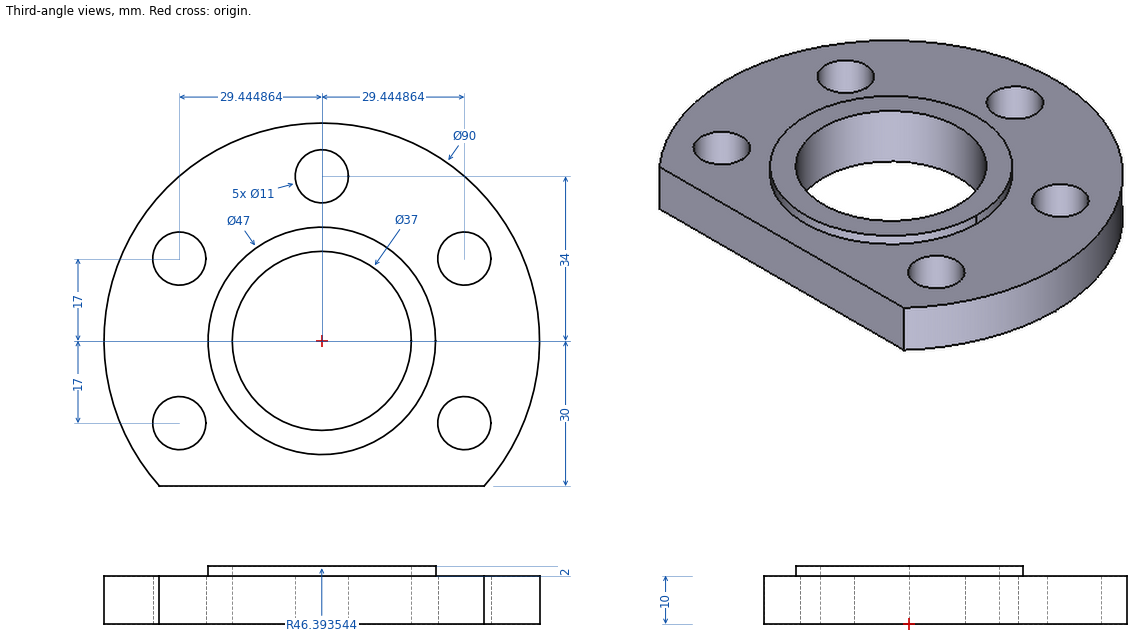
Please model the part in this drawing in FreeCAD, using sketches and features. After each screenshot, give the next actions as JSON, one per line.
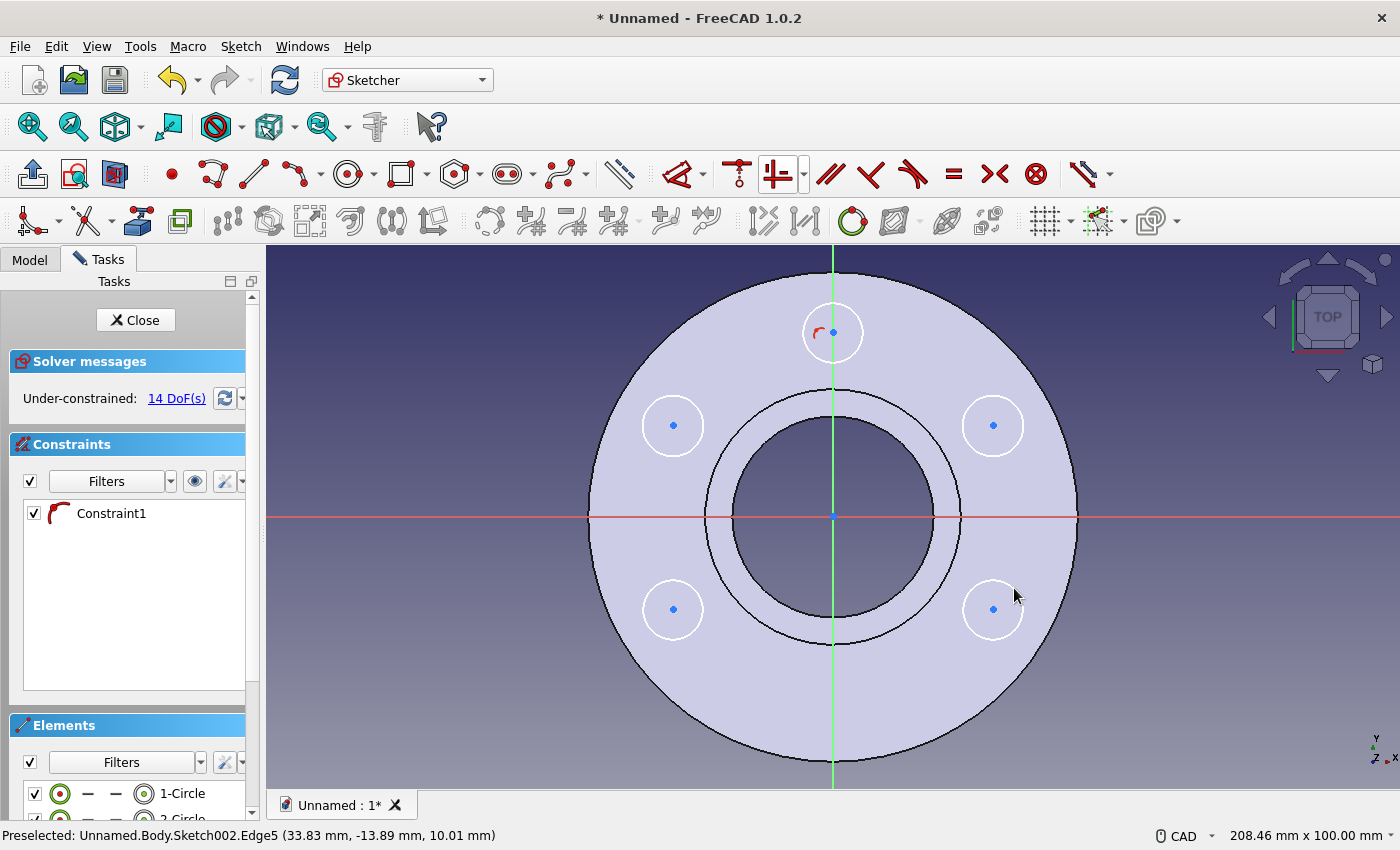
{"action": "left_click", "coordinate": [854, 312]}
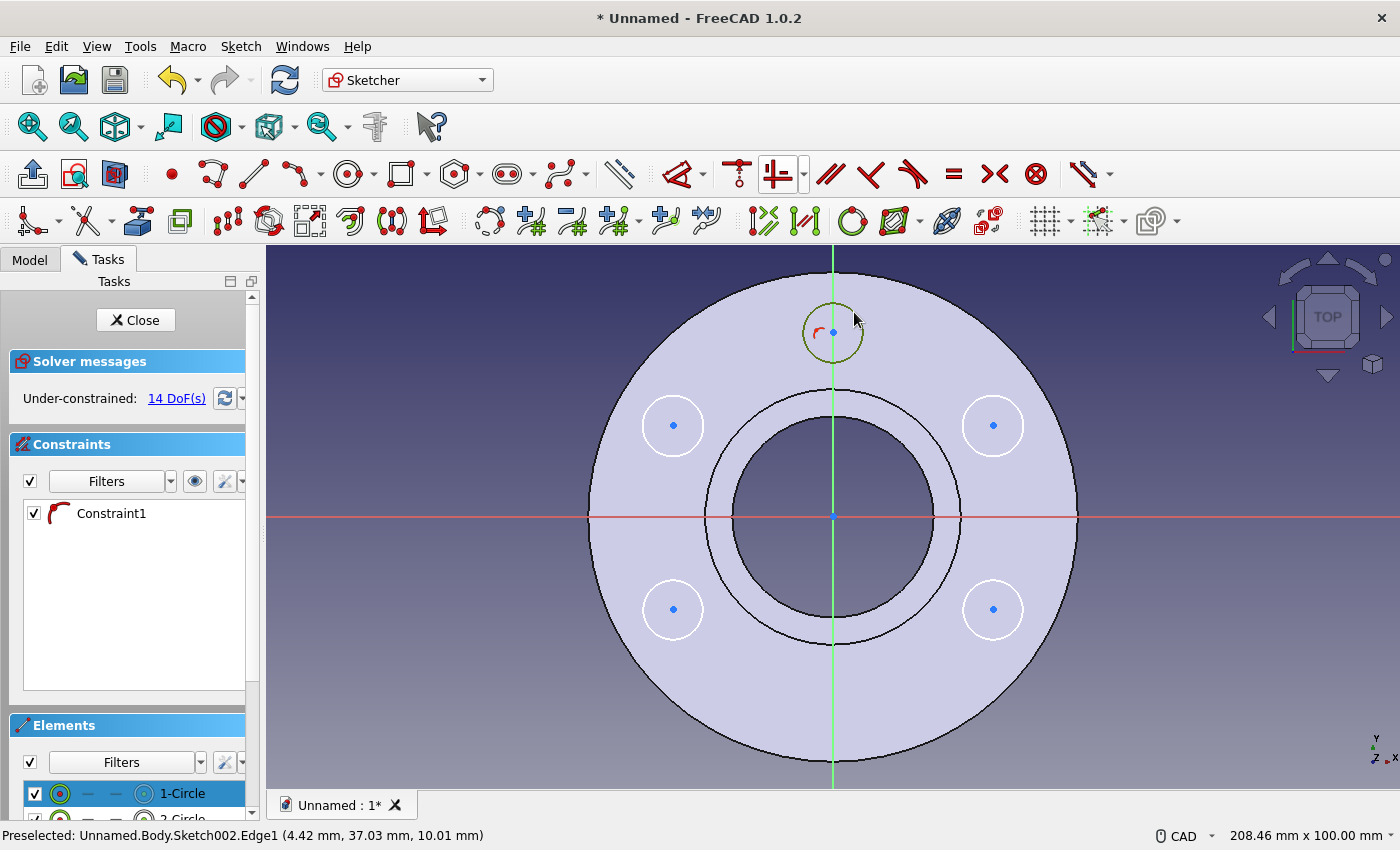
{"action": "left_click", "coordinate": [694, 404]}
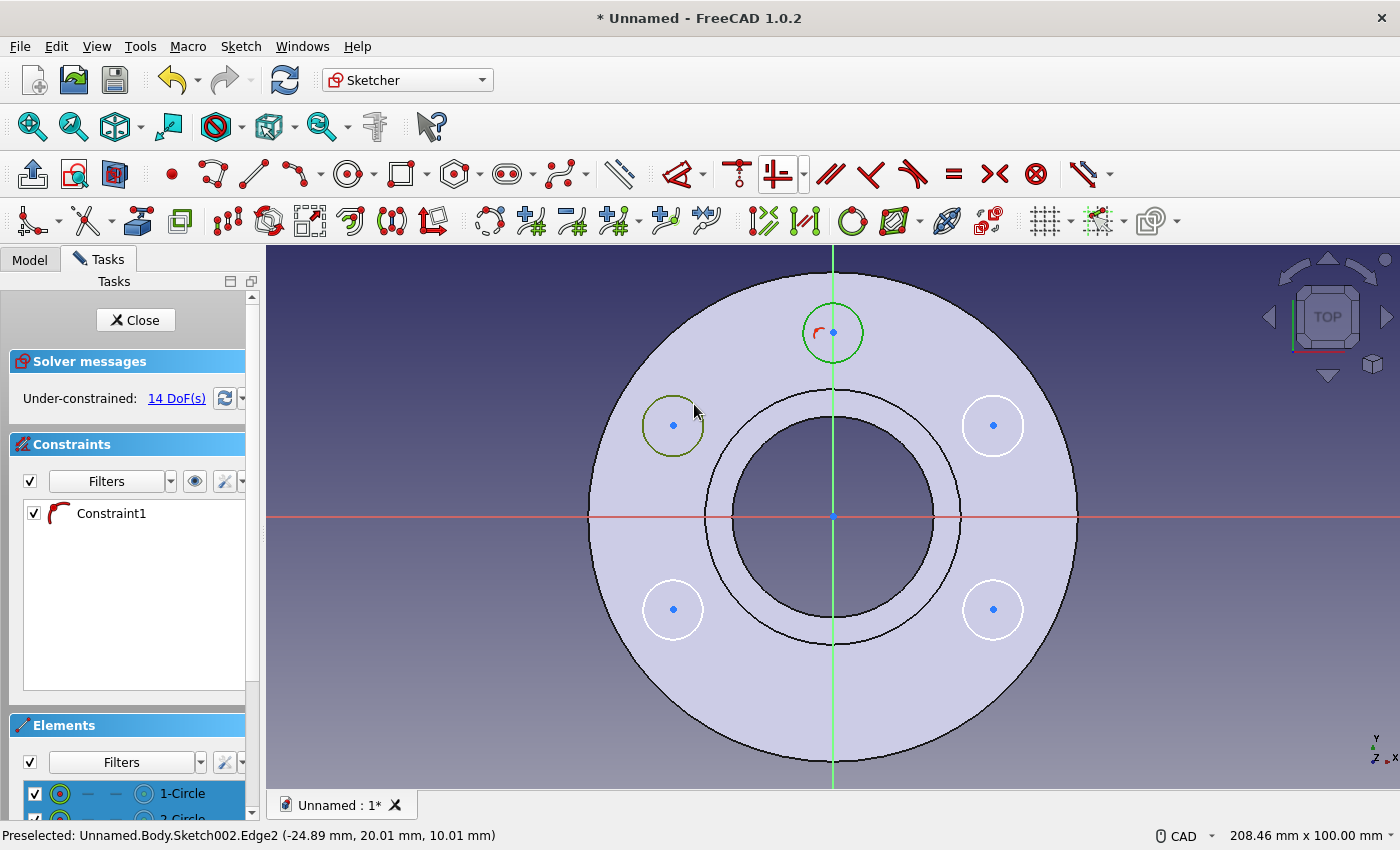
{"action": "left_click", "coordinate": [694, 589]}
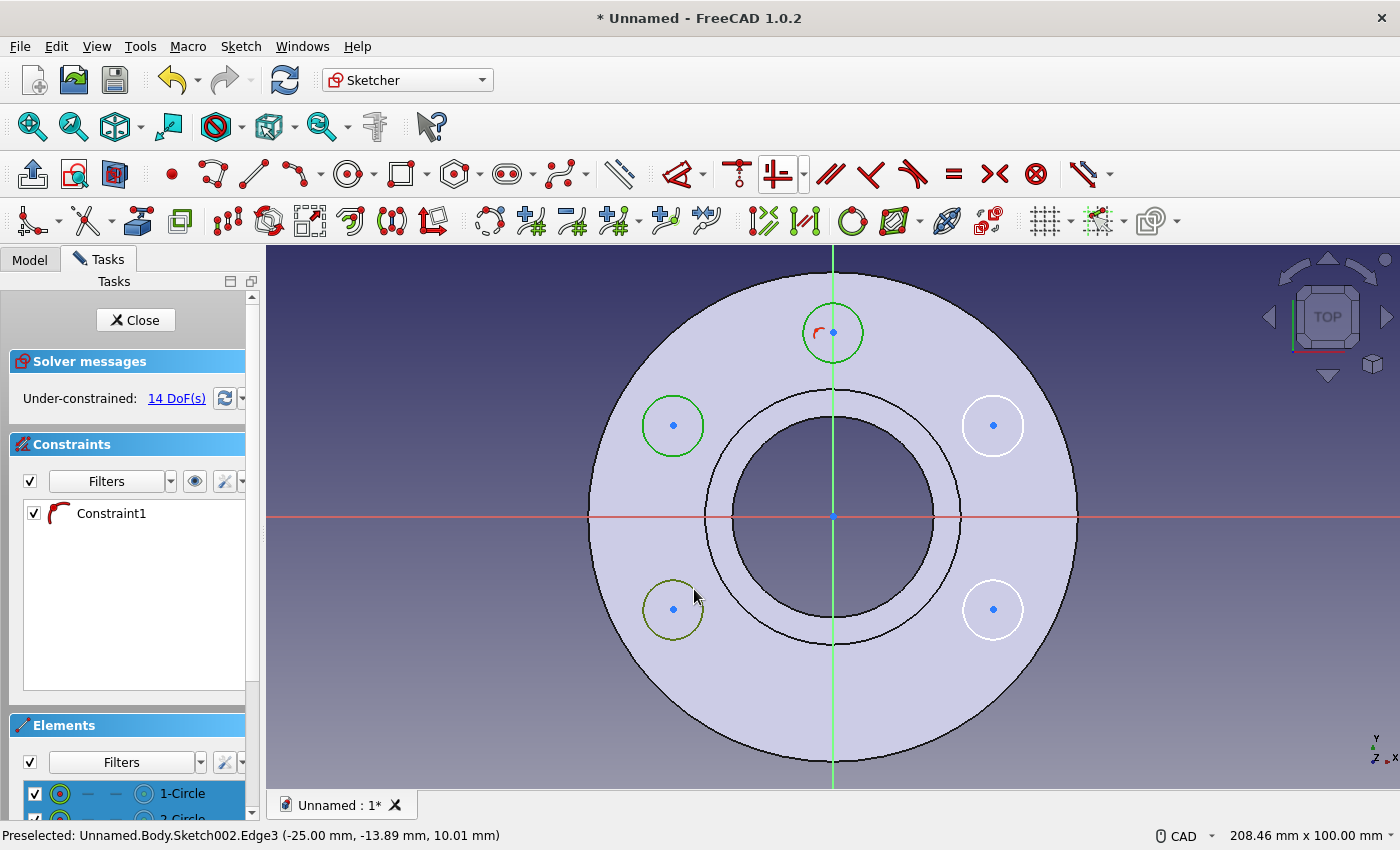
{"action": "left_click", "coordinate": [1014, 404]}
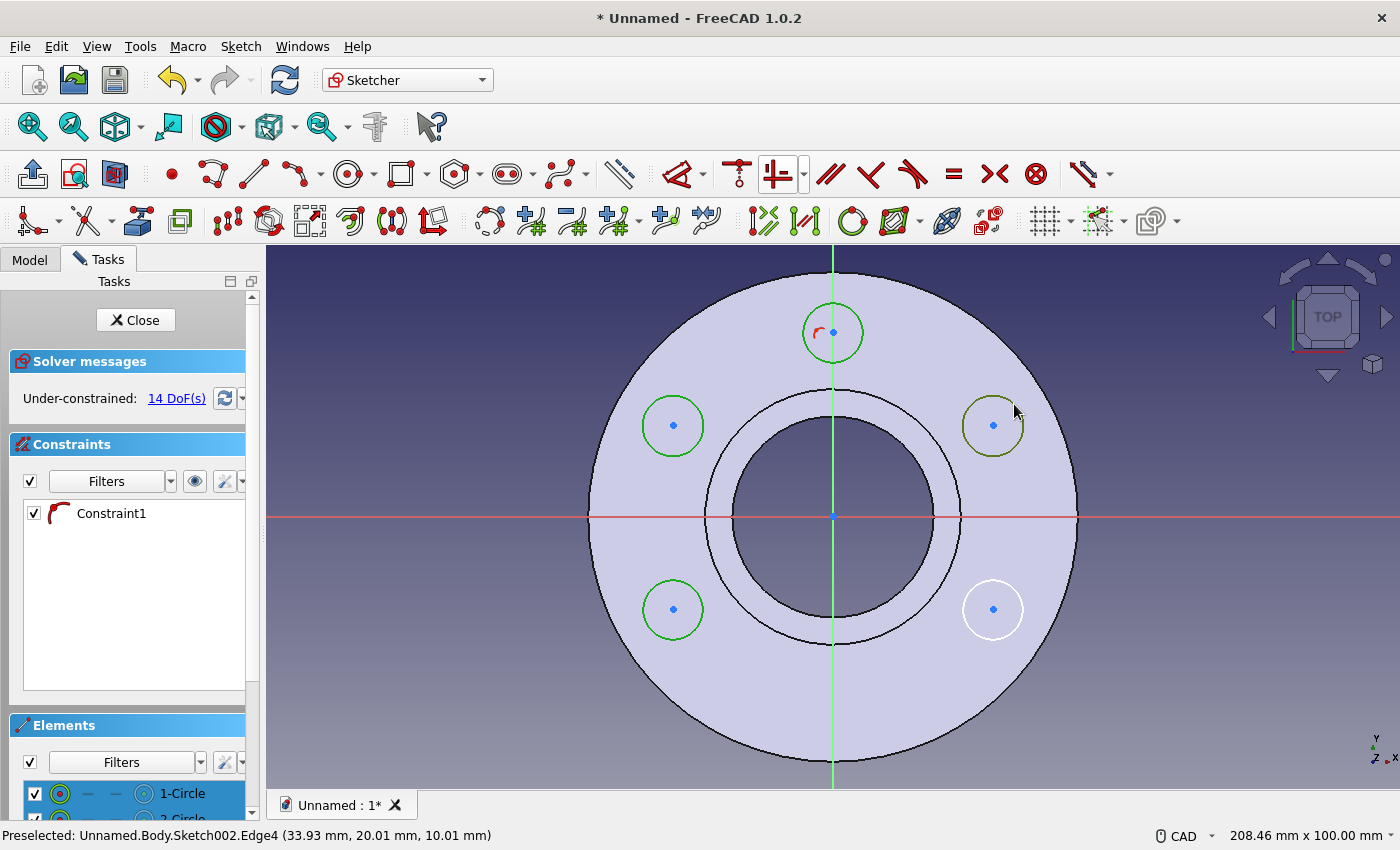
{"action": "left_click", "coordinate": [1014, 589]}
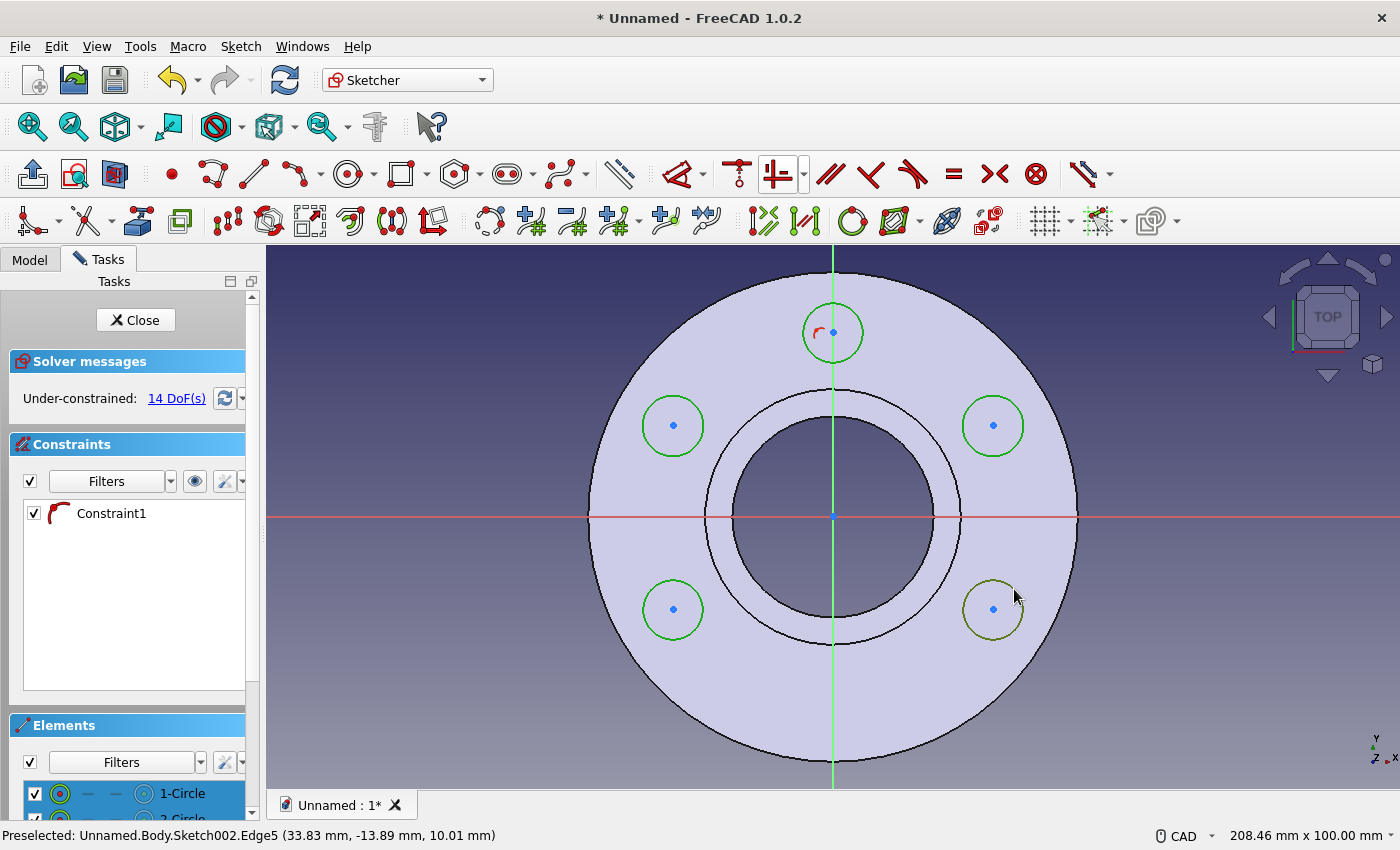
{"action": "left_click", "coordinate": [954, 174]}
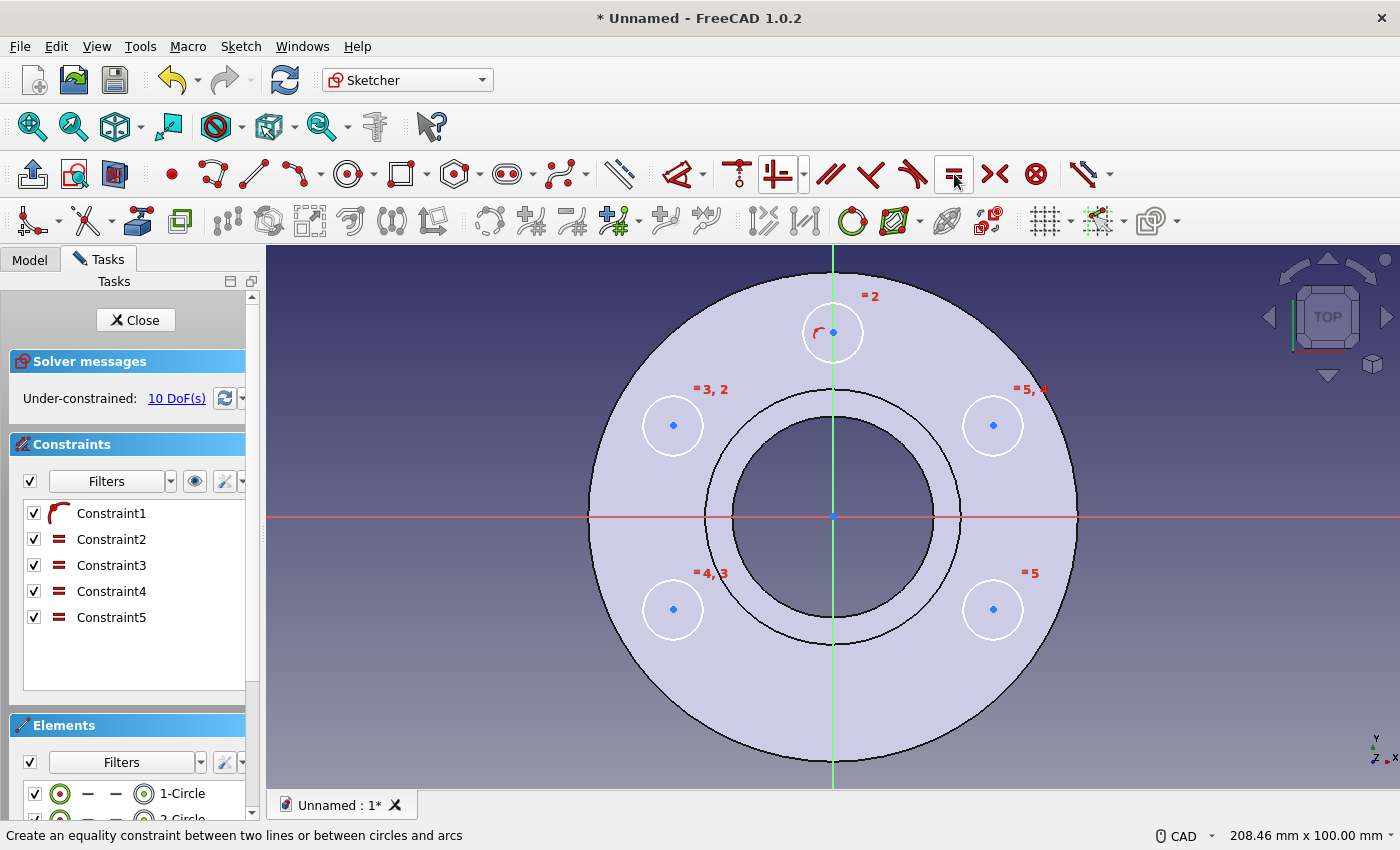
{"action": "left_click", "coordinate": [673, 426]}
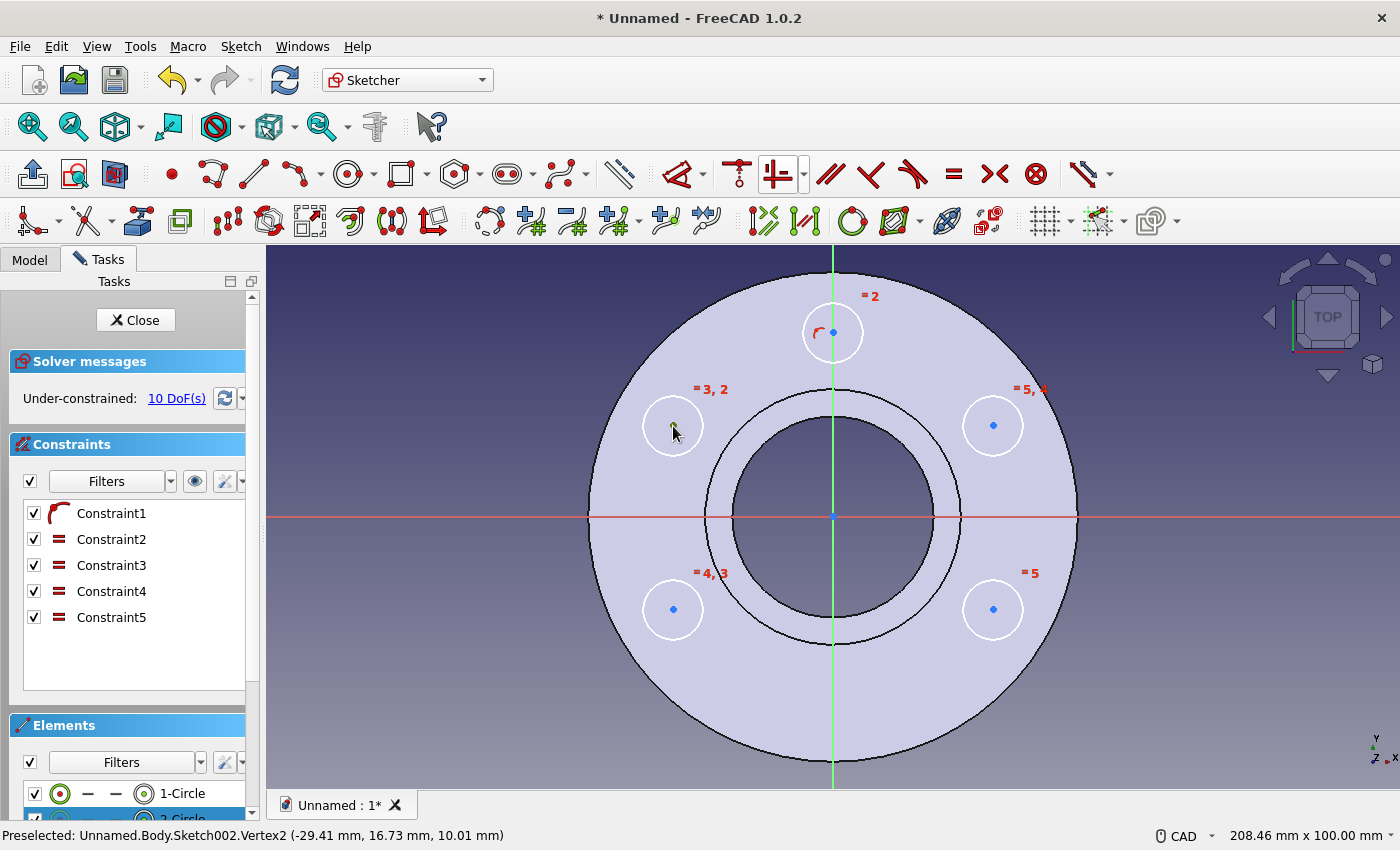
{"action": "left_click", "coordinate": [673, 610]}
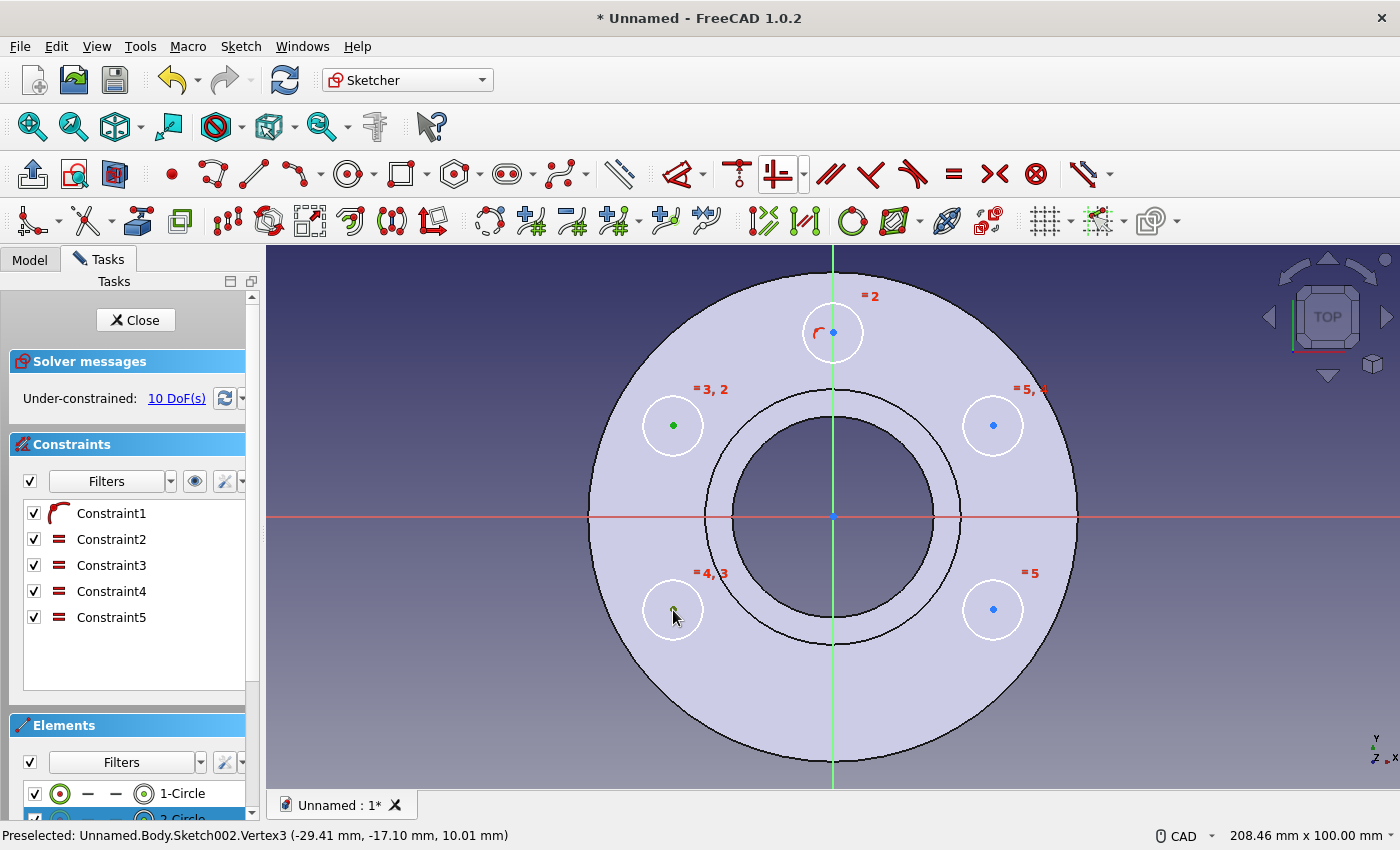
{"action": "left_click", "coordinate": [804, 174]}